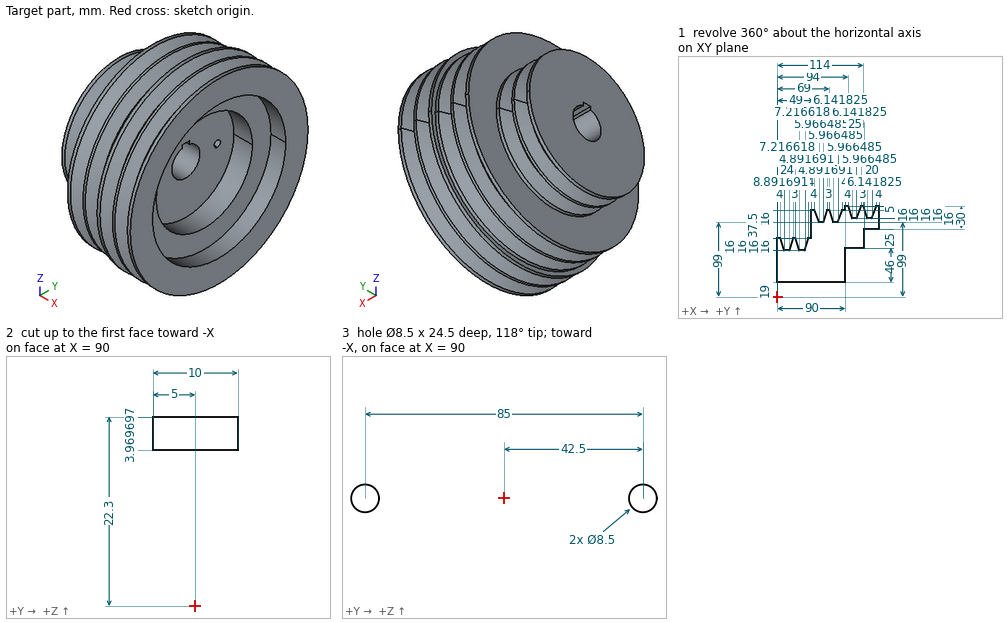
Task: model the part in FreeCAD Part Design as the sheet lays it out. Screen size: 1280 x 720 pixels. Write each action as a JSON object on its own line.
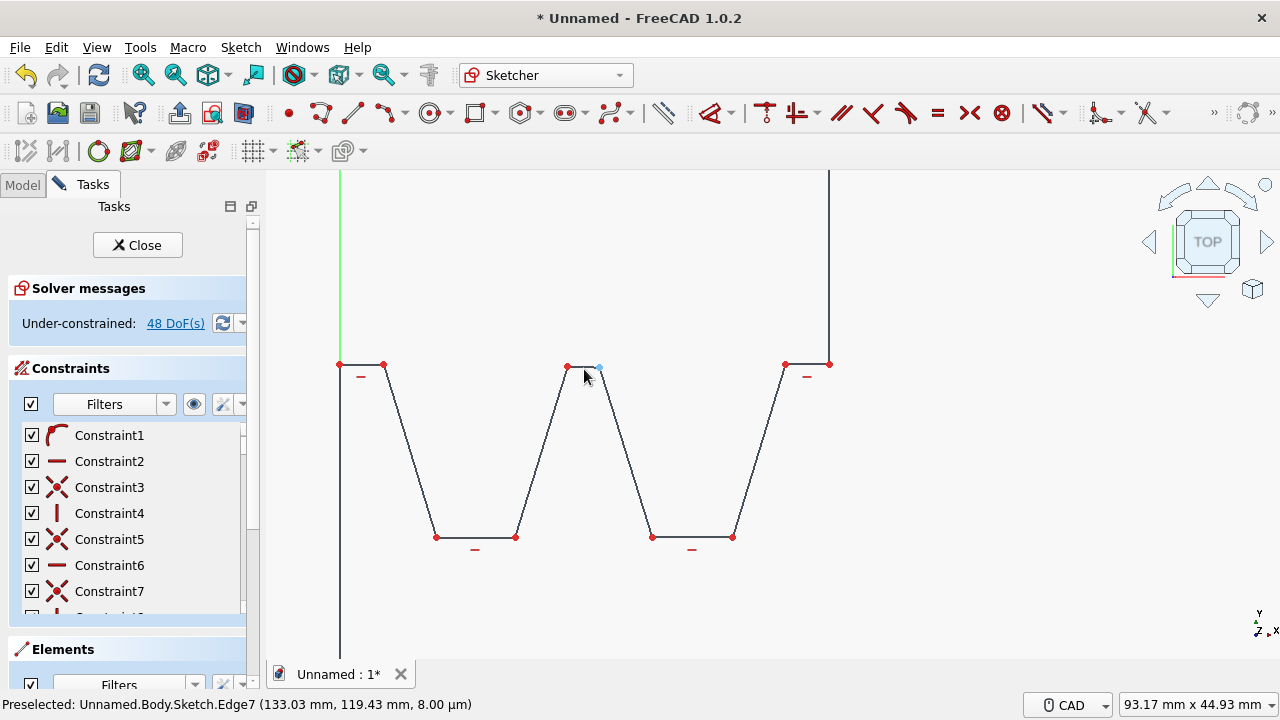
{"action": "left_click", "coordinate": [584, 367]}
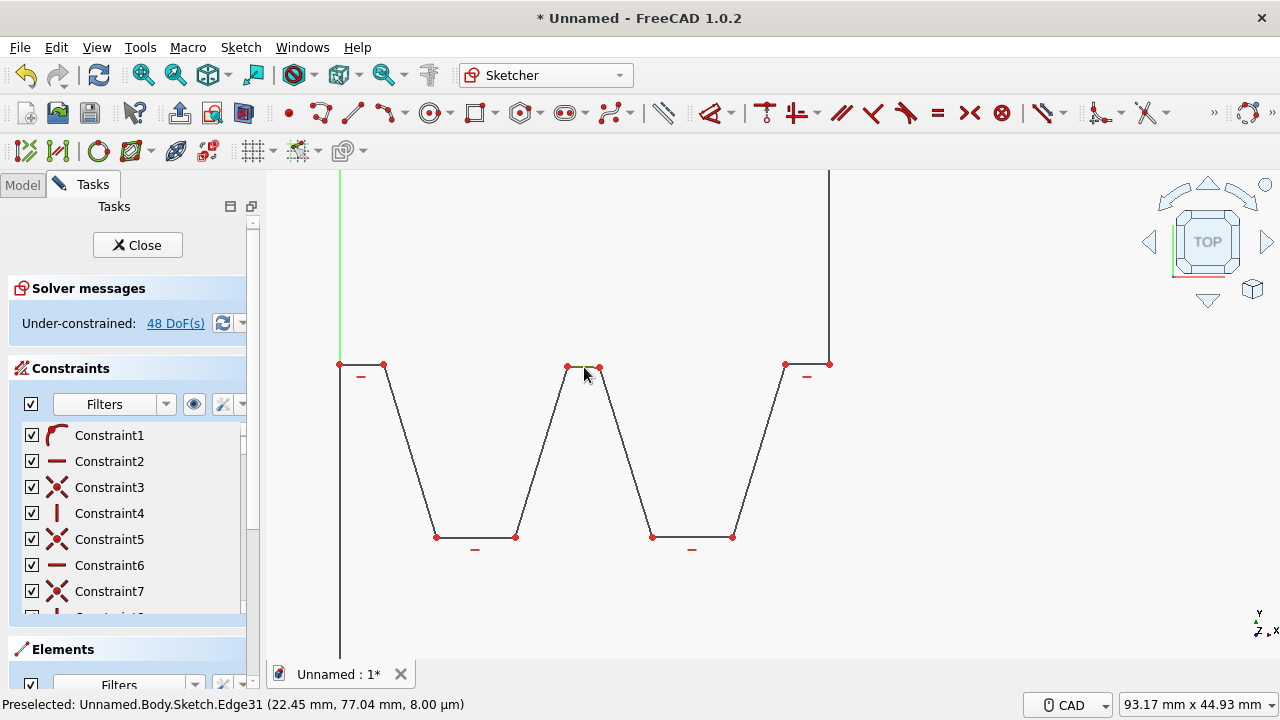
{"action": "key", "text": "h"}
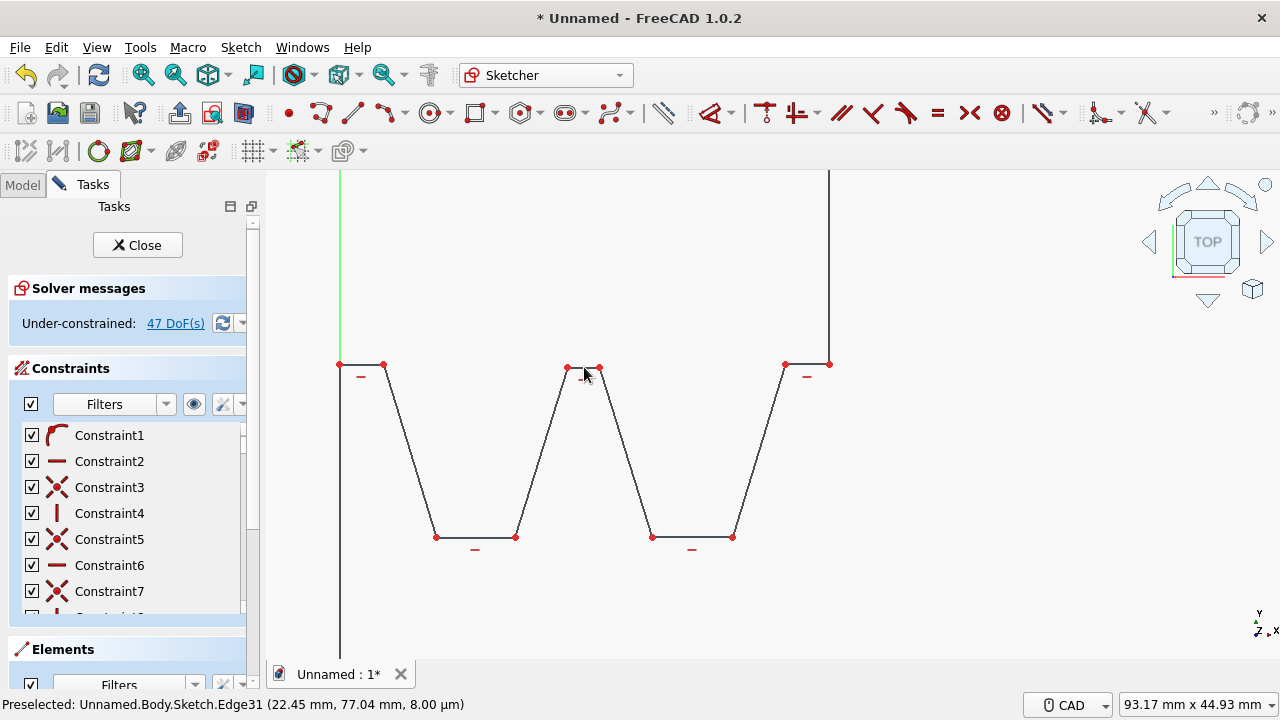
{"action": "key", "text": "d"}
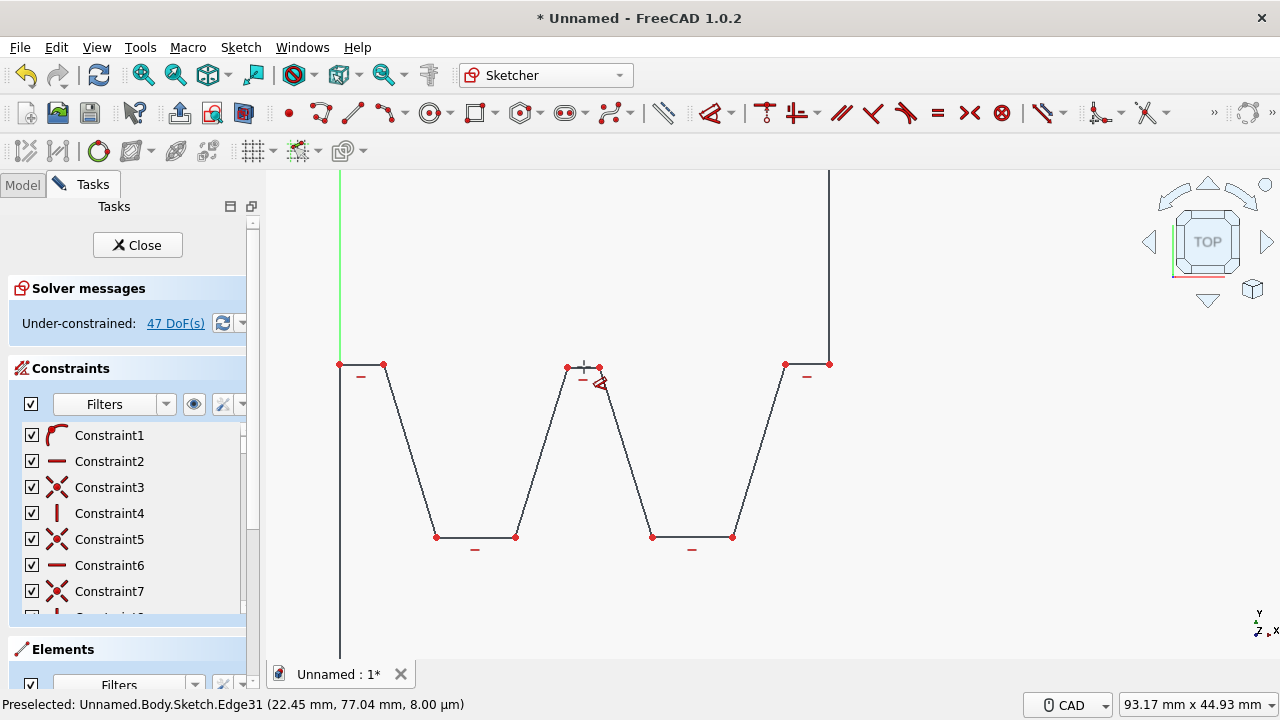
{"action": "scroll", "coordinate": [583, 369], "scroll_direction": "down", "scroll_amount": 7}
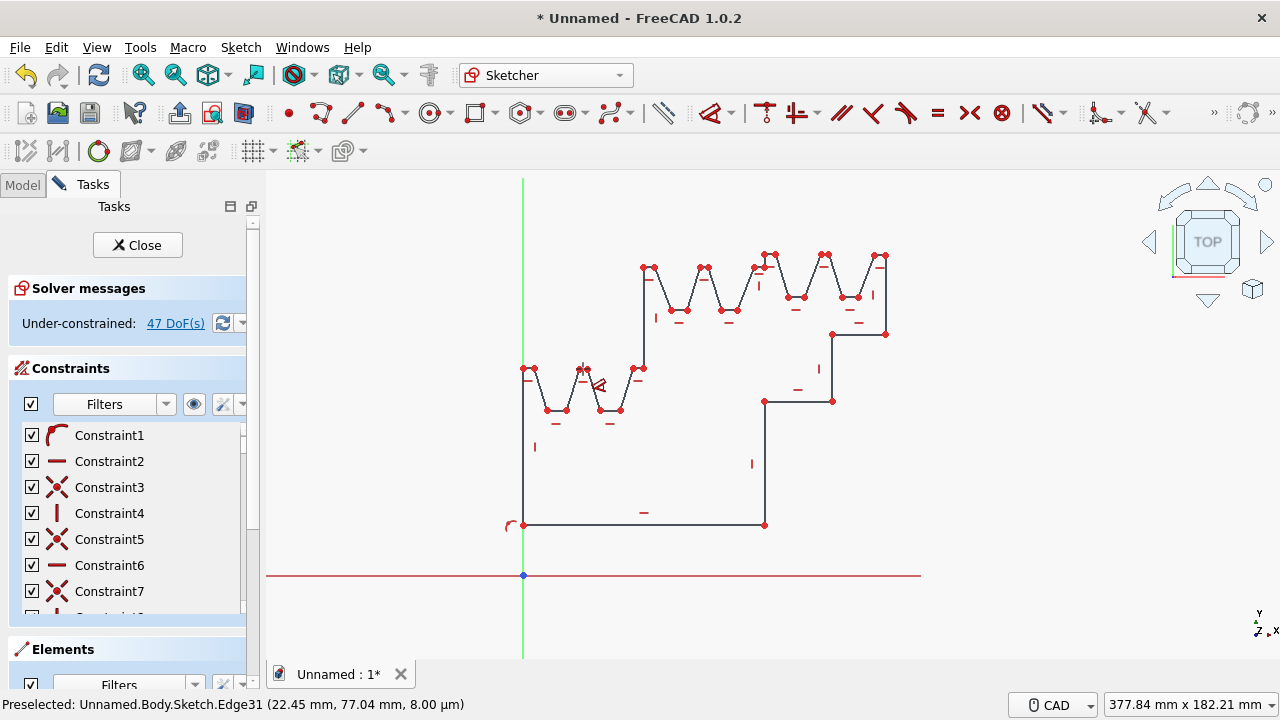
{"action": "scroll", "coordinate": [882, 255], "scroll_direction": "up", "scroll_amount": 8}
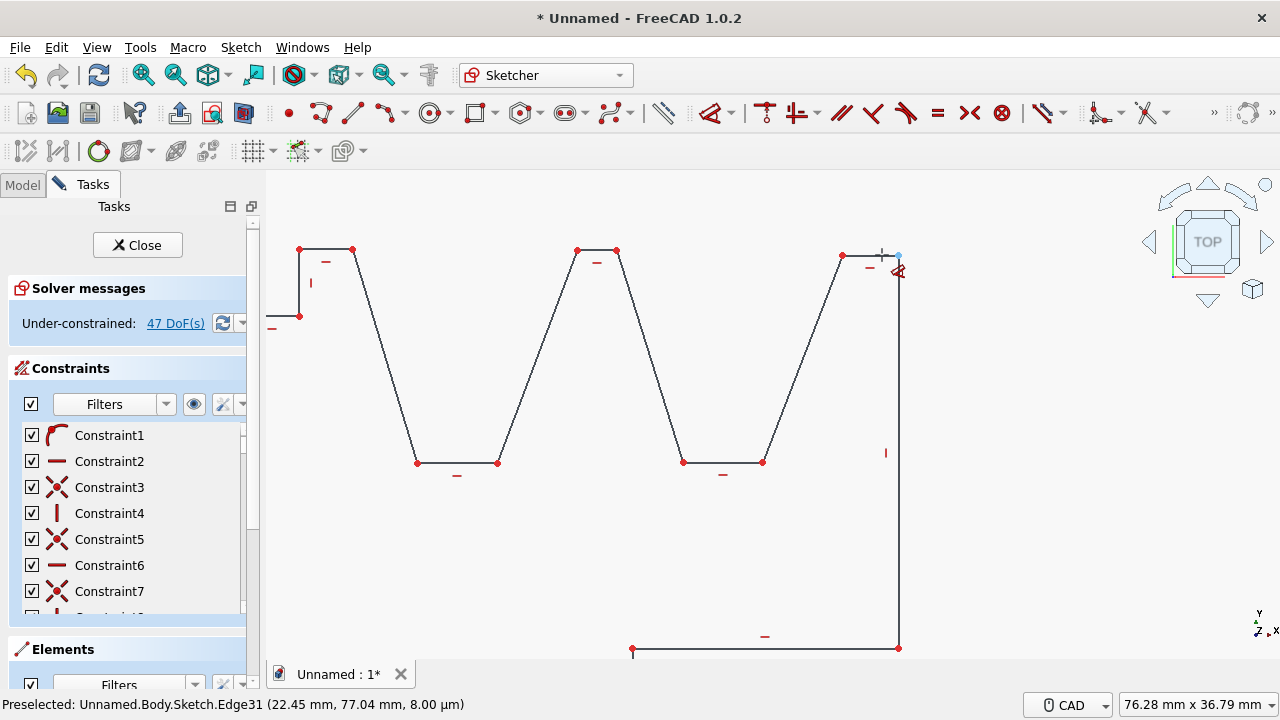
{"action": "left_click", "coordinate": [882, 256]}
{"action": "left_click", "coordinate": [871, 222]}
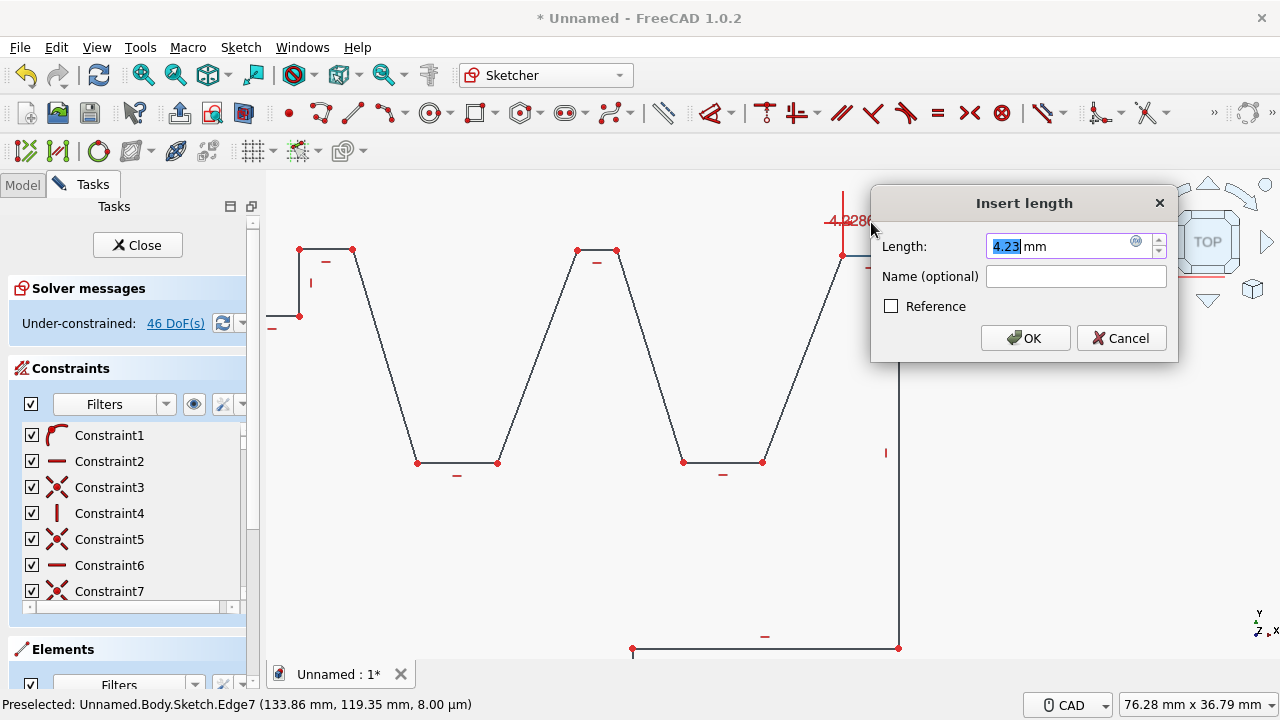
{"action": "type", "text": "4"}
{"action": "key", "text": "Return"}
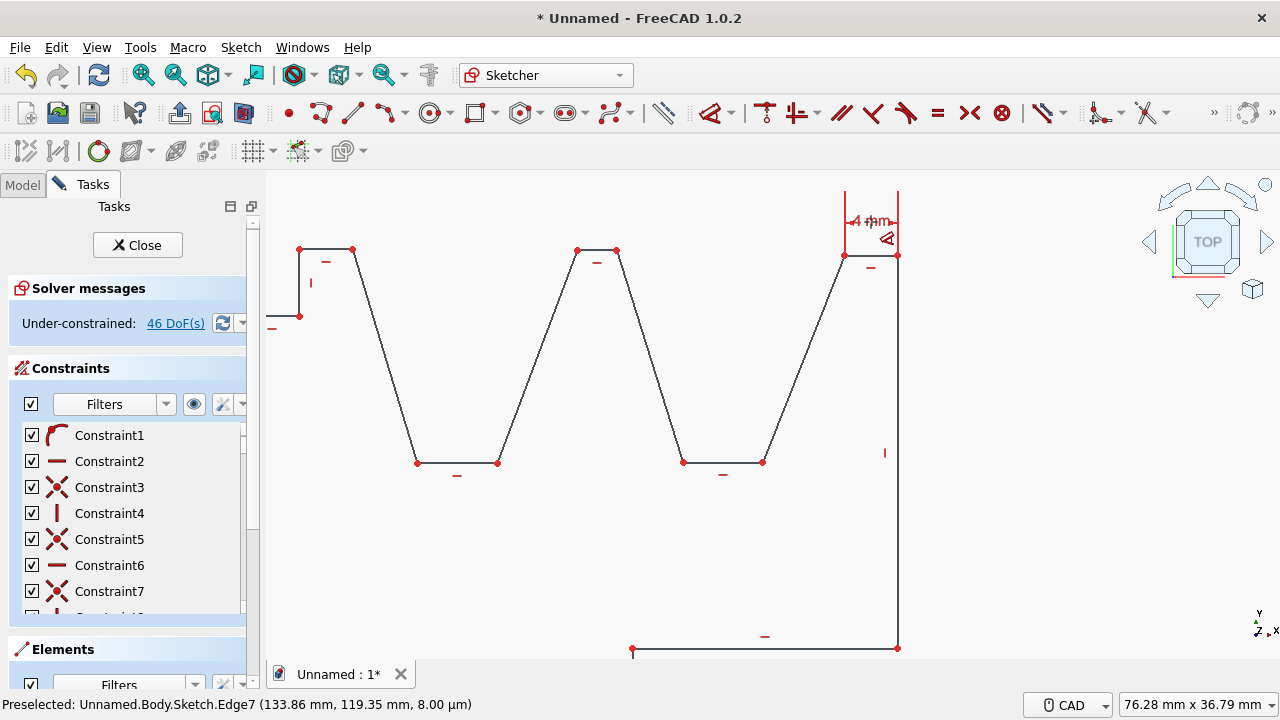
{"action": "left_click", "coordinate": [605, 250]}
{"action": "left_click", "coordinate": [597, 216]}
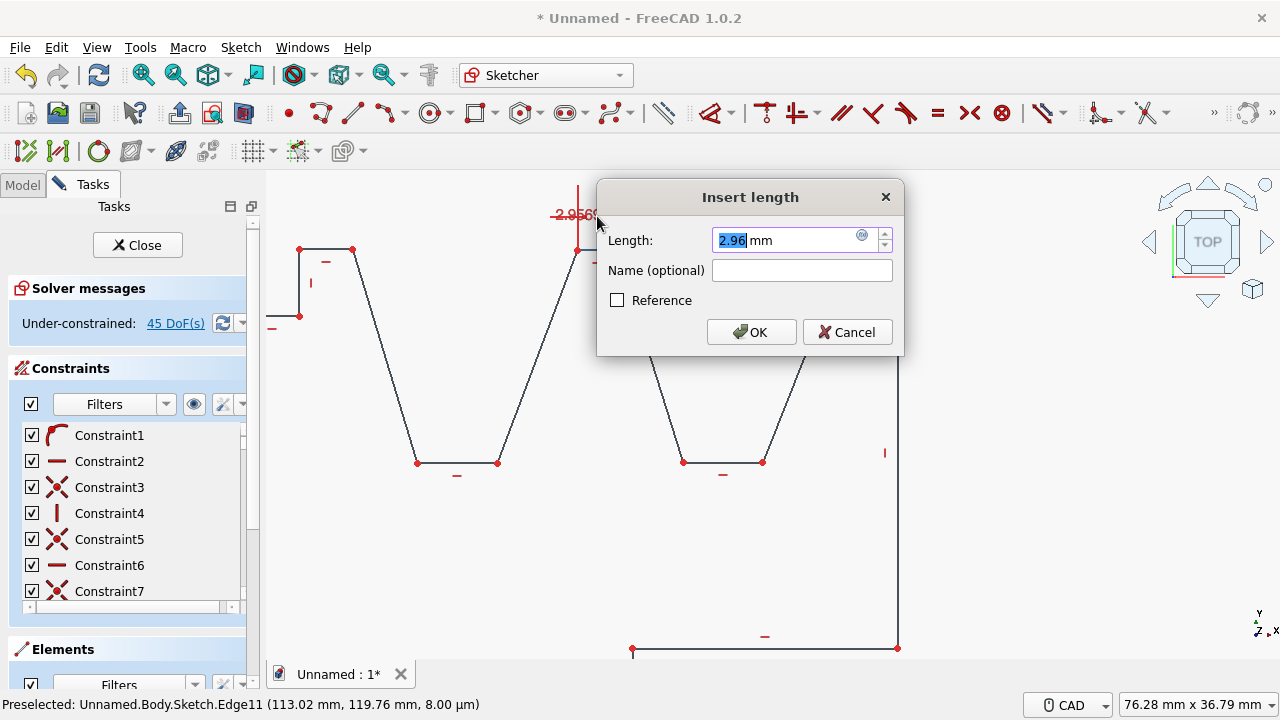
{"action": "type", "text": "3"}
{"action": "key", "text": "Return"}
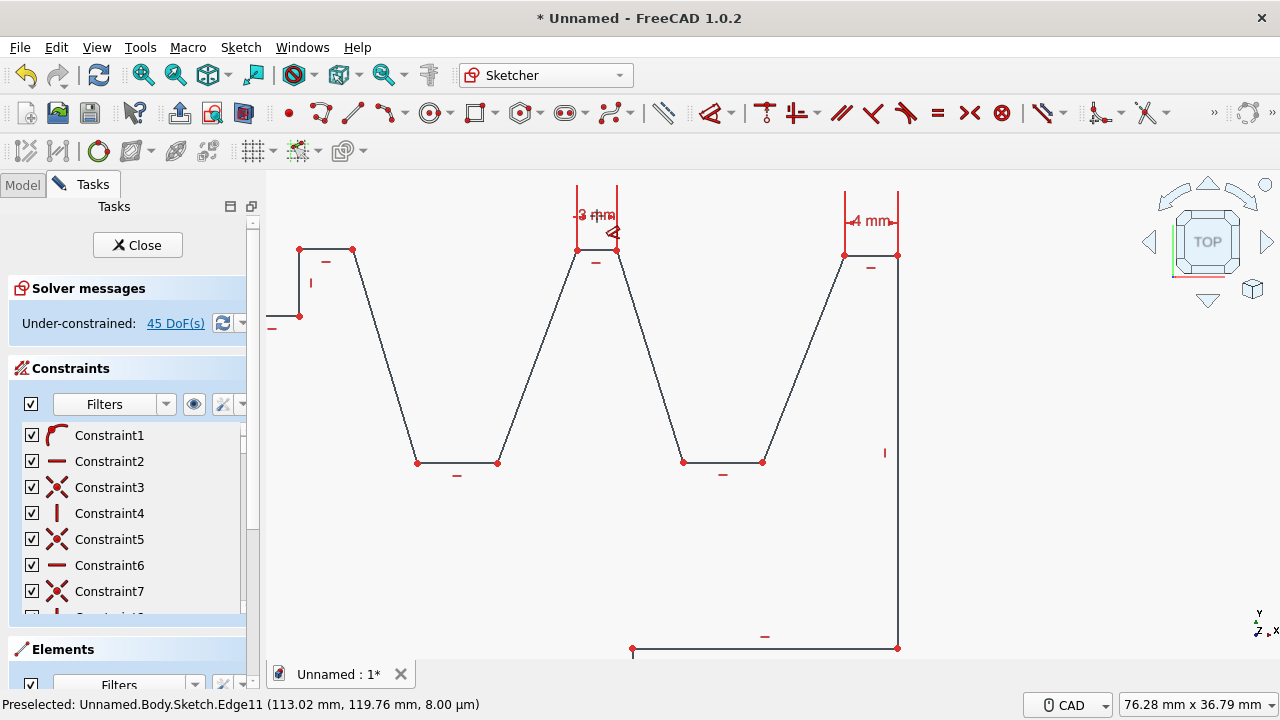
{"action": "left_click", "coordinate": [337, 249]}
{"action": "left_click", "coordinate": [326, 215]}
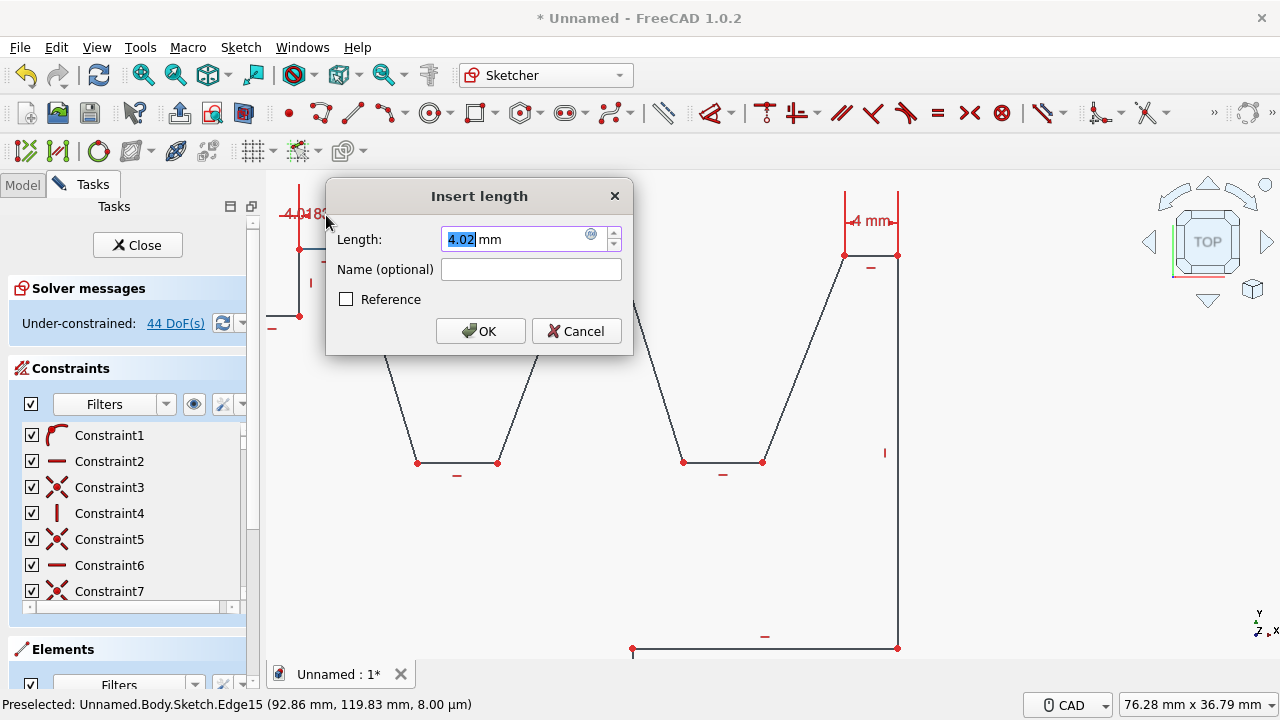
{"action": "type", "text": "4"}
{"action": "key", "text": "Return"}